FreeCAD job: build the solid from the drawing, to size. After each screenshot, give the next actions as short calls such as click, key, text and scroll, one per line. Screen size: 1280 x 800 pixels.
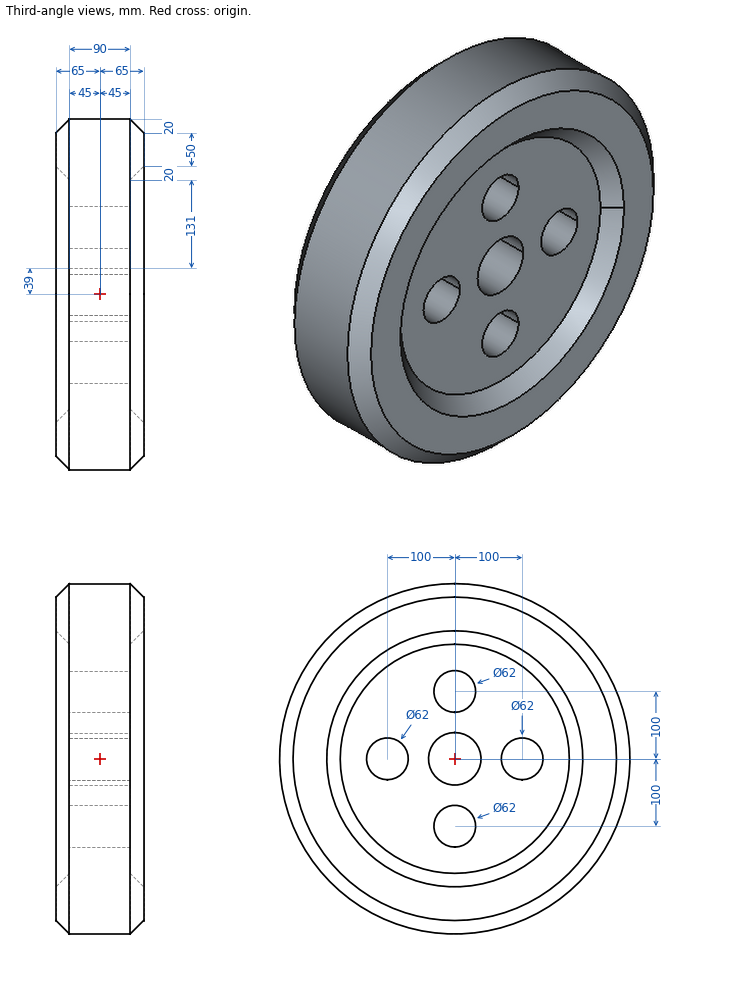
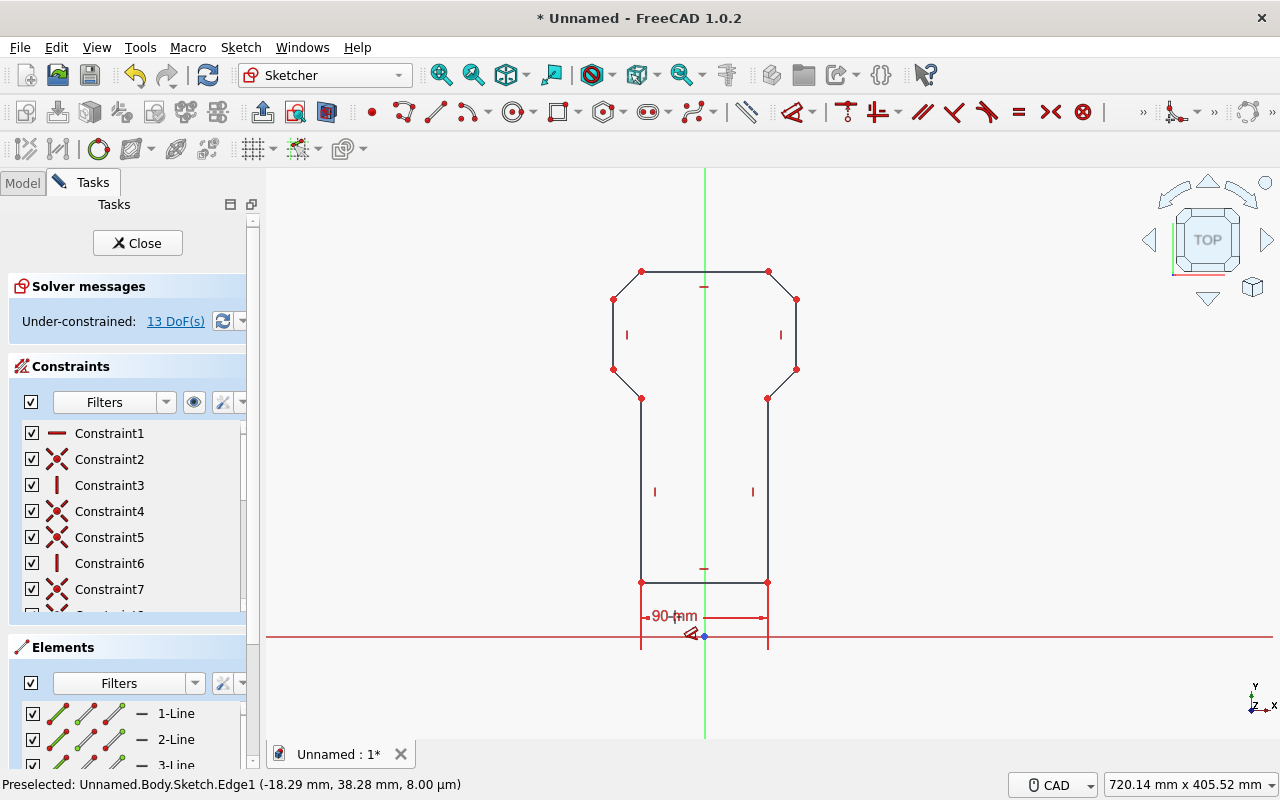
click(796, 349)
click(830, 335)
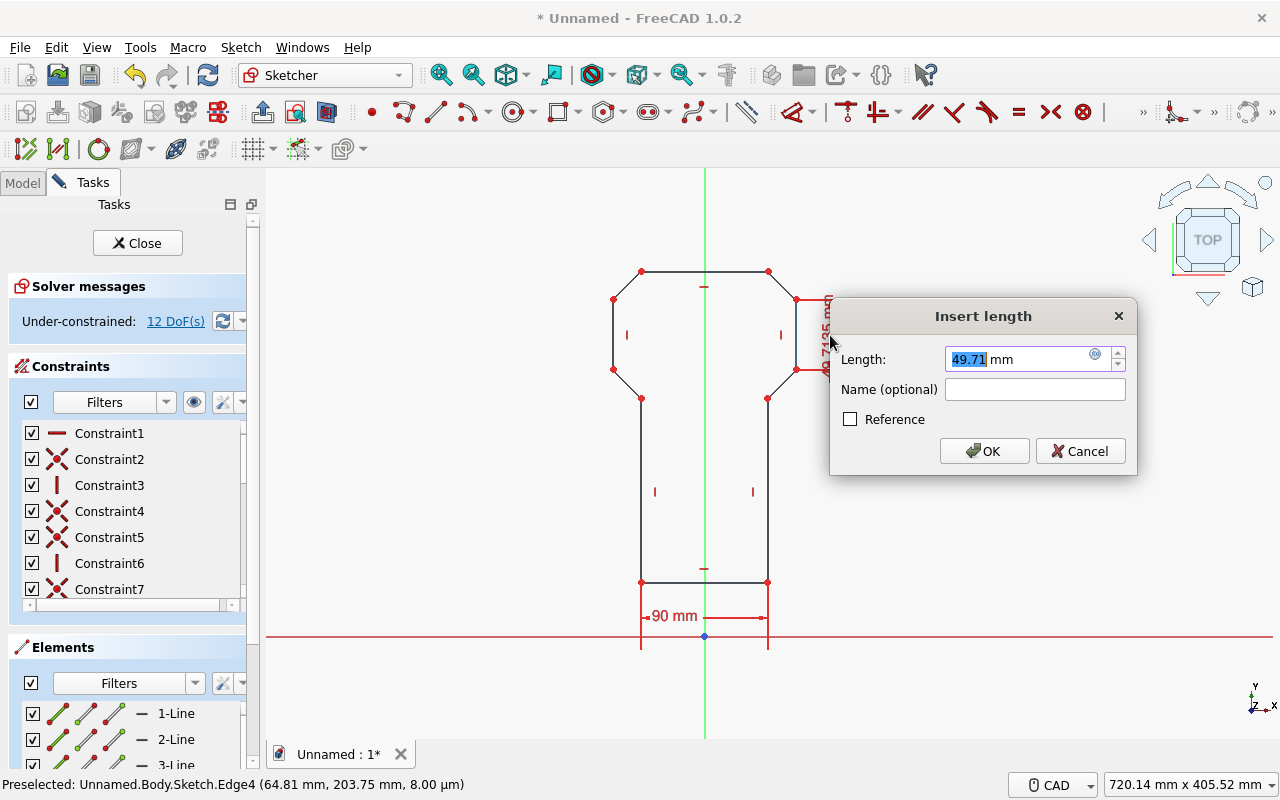
text(50)
key(Return)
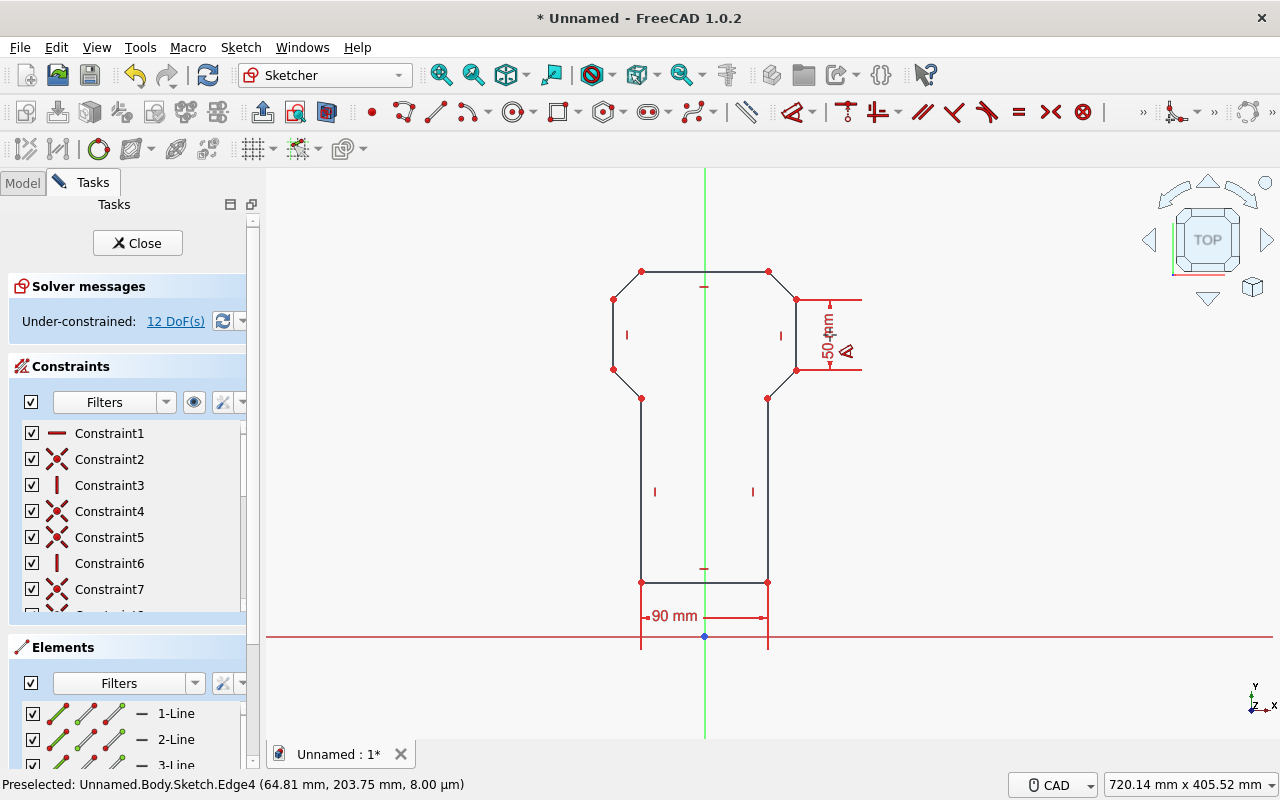
click(730, 272)
click(675, 238)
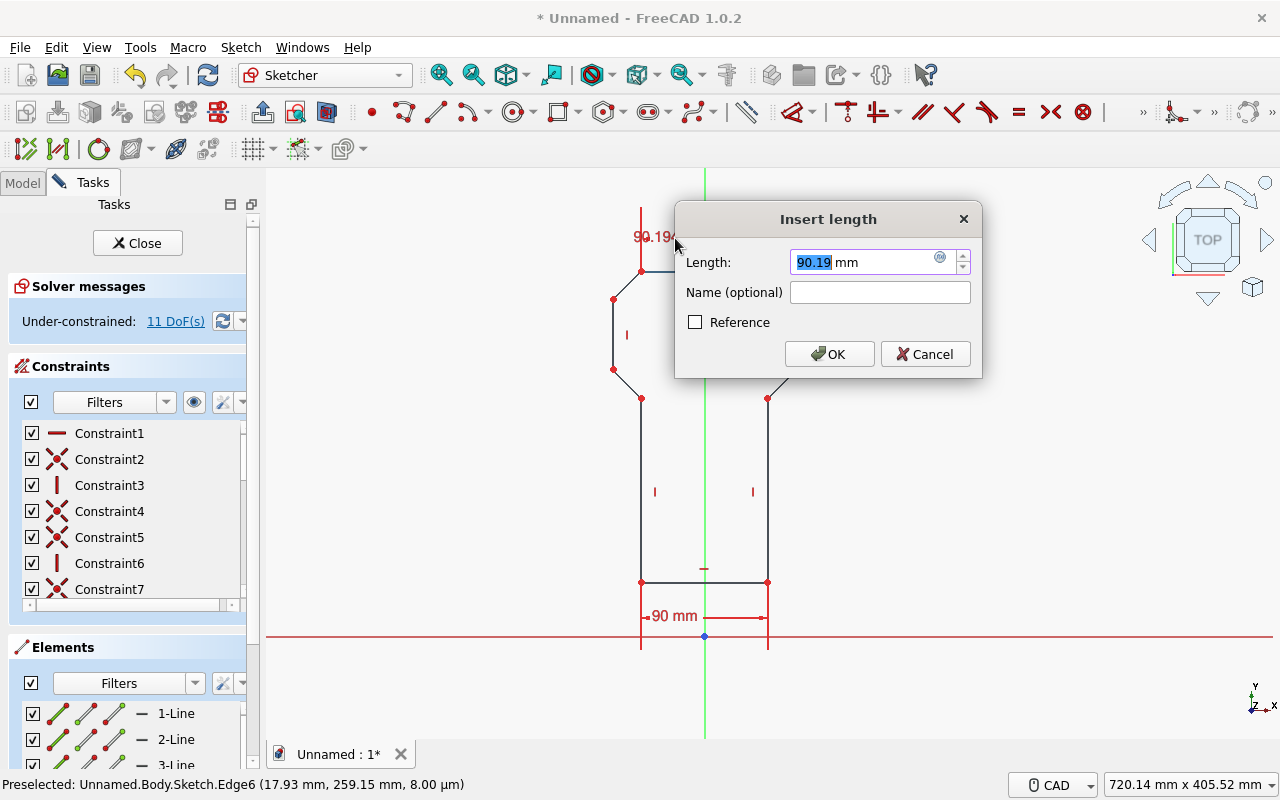
text(90)
key(Return)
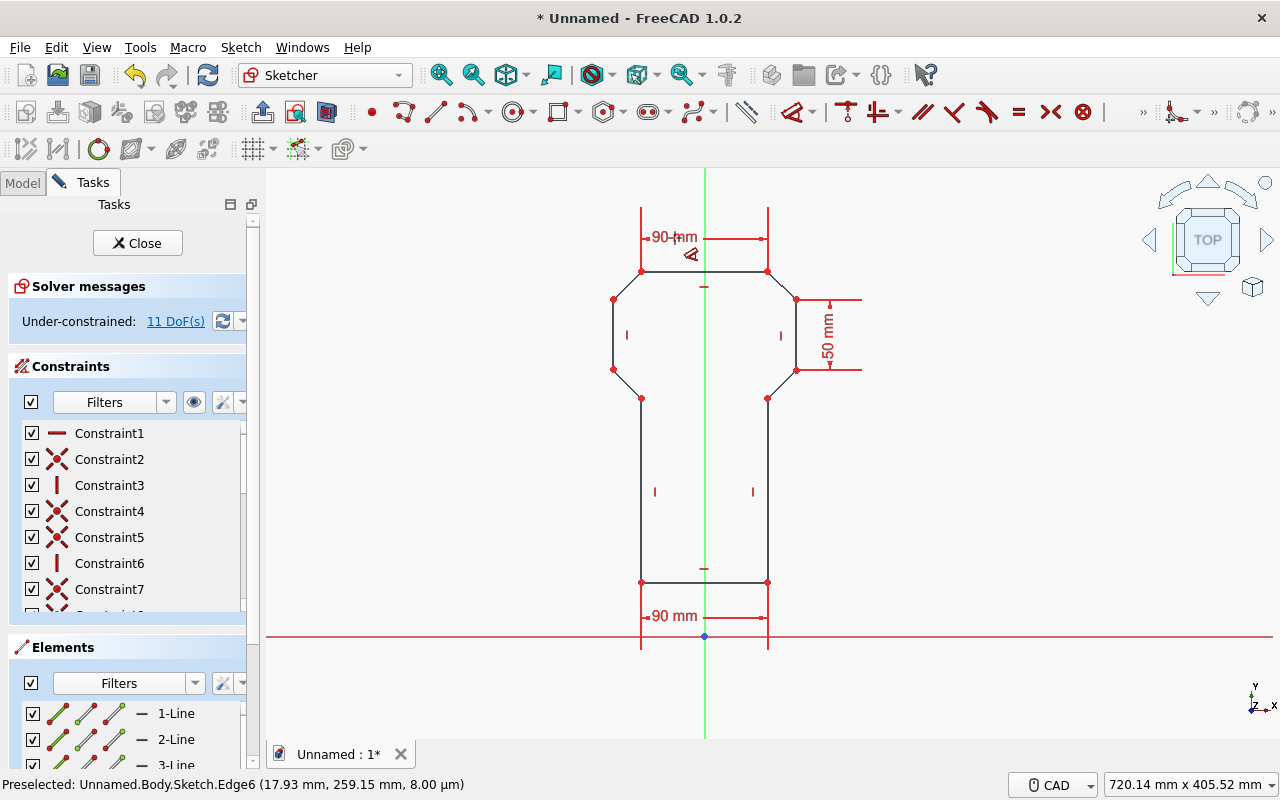
click(613, 321)
click(579, 335)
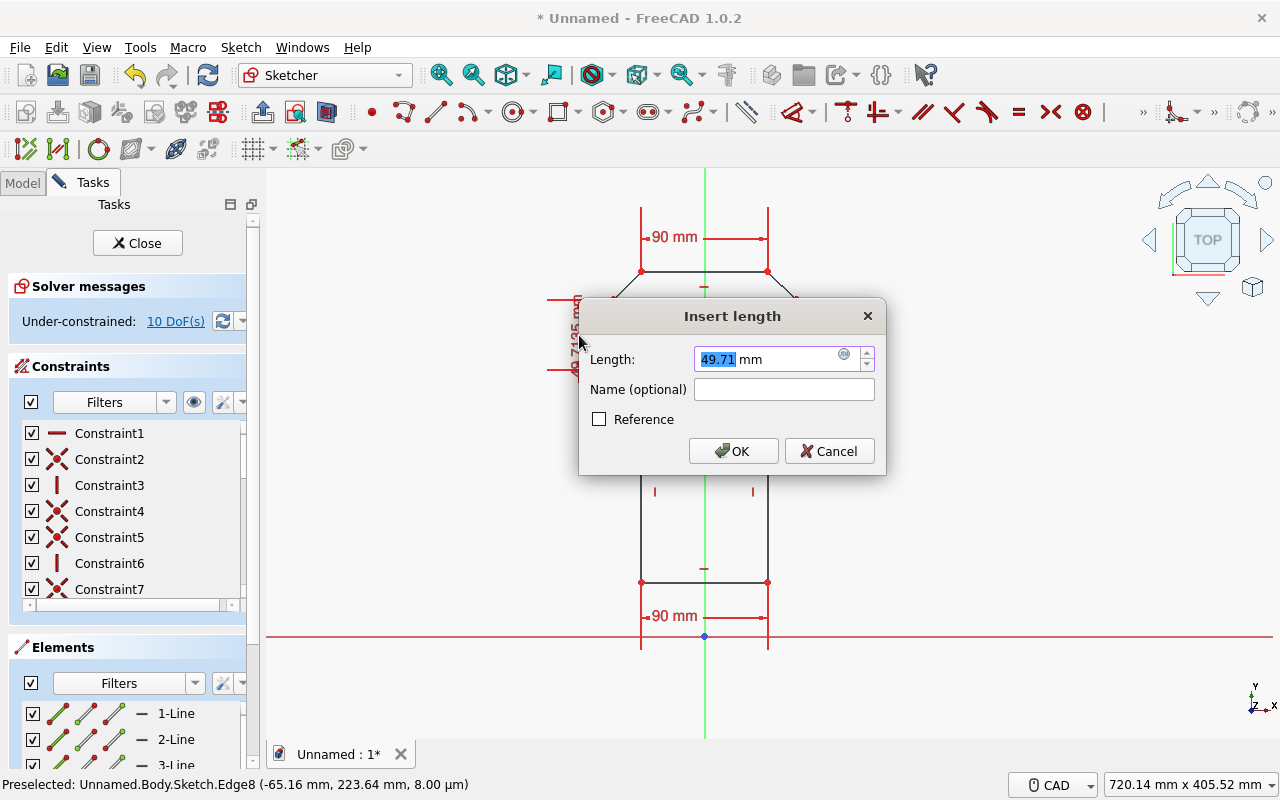
text(50)
key(Return)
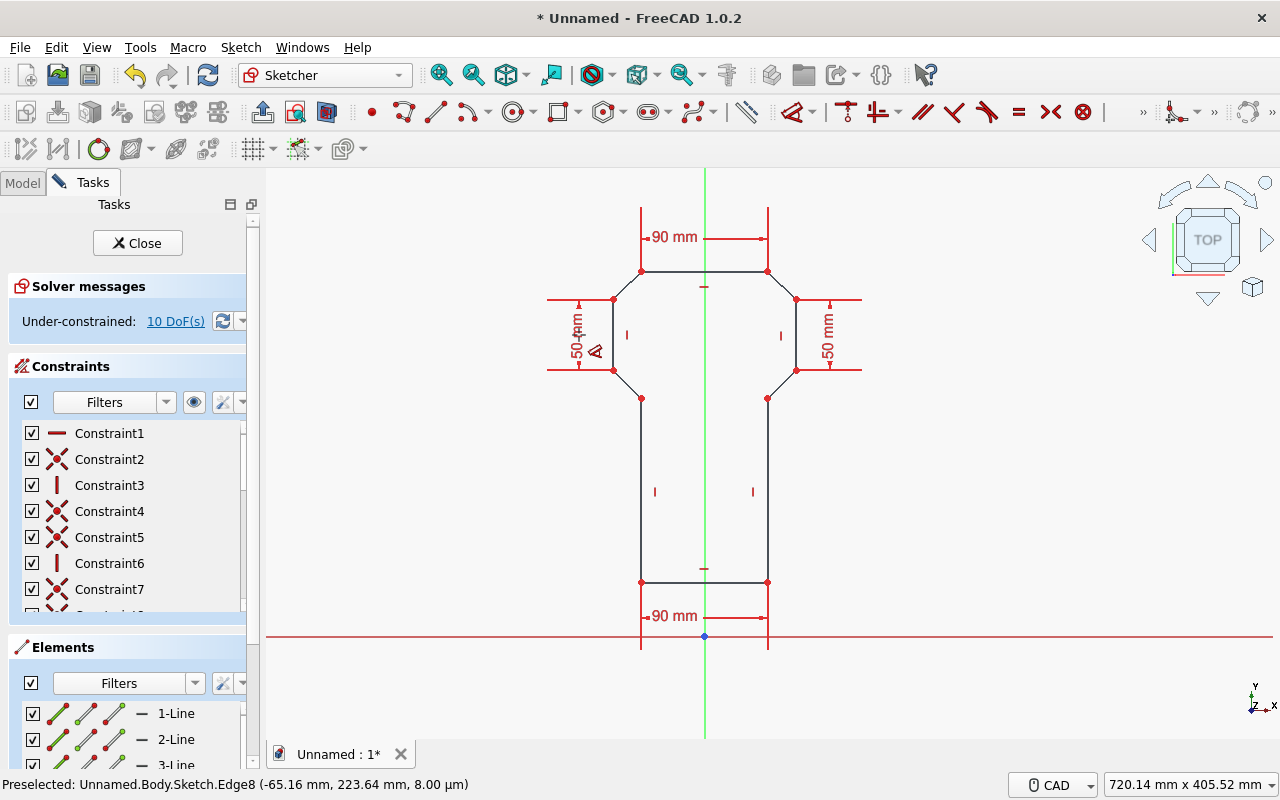
click(768, 528)
click(802, 491)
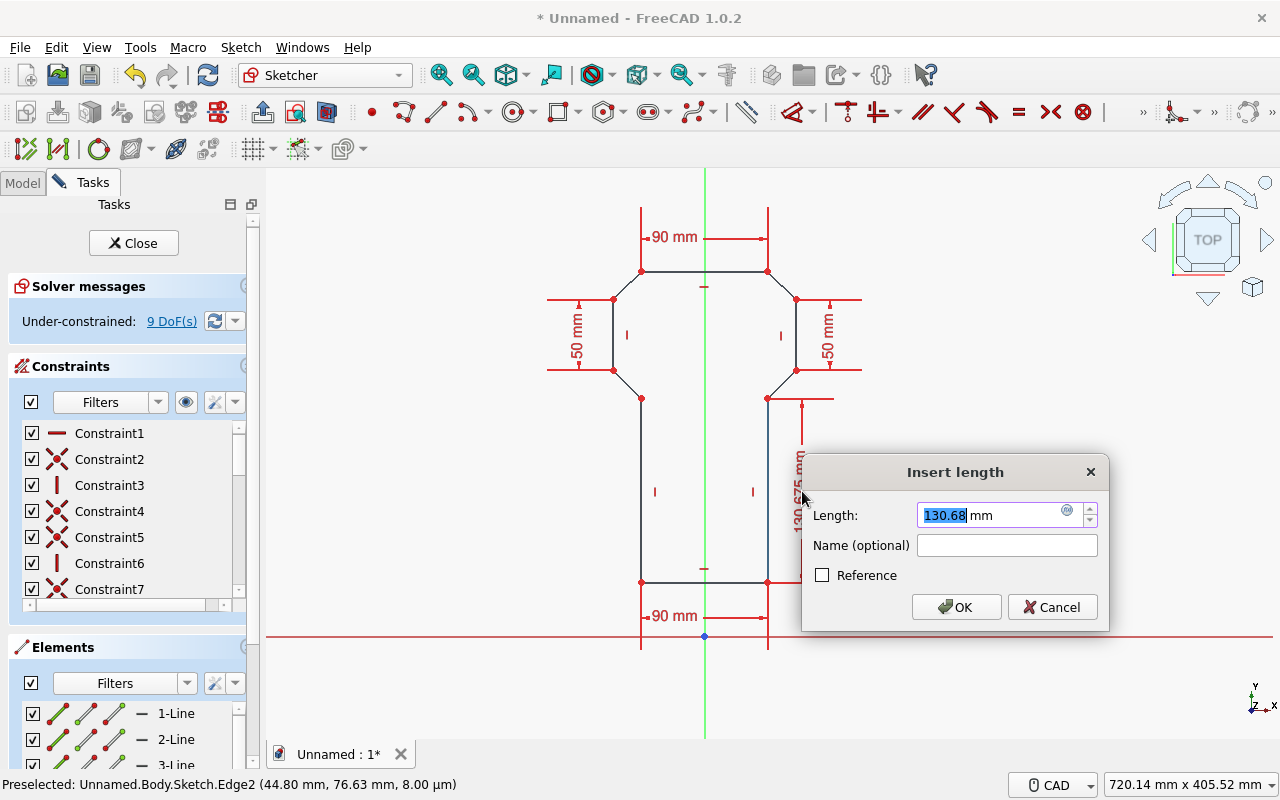
text(131)
key(Return)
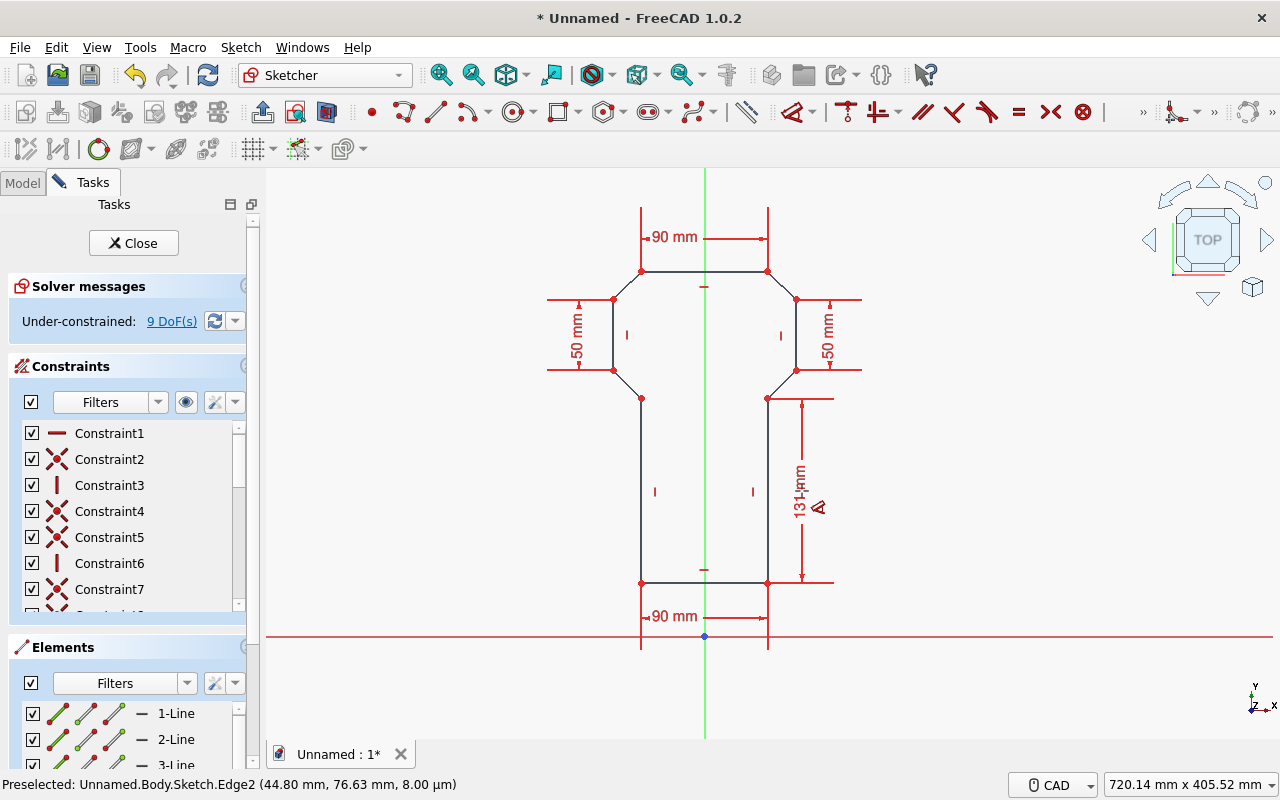
click(641, 454)
click(607, 491)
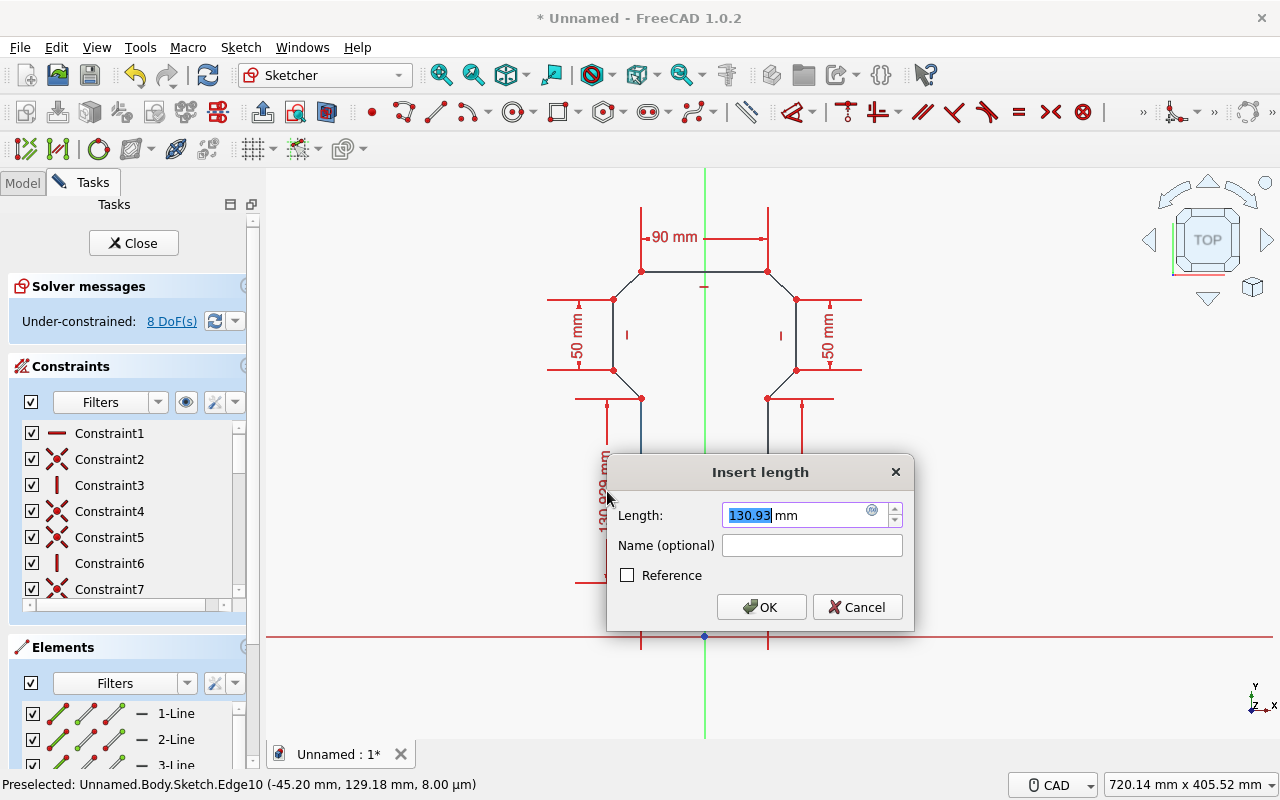
text(131)
key(Return)